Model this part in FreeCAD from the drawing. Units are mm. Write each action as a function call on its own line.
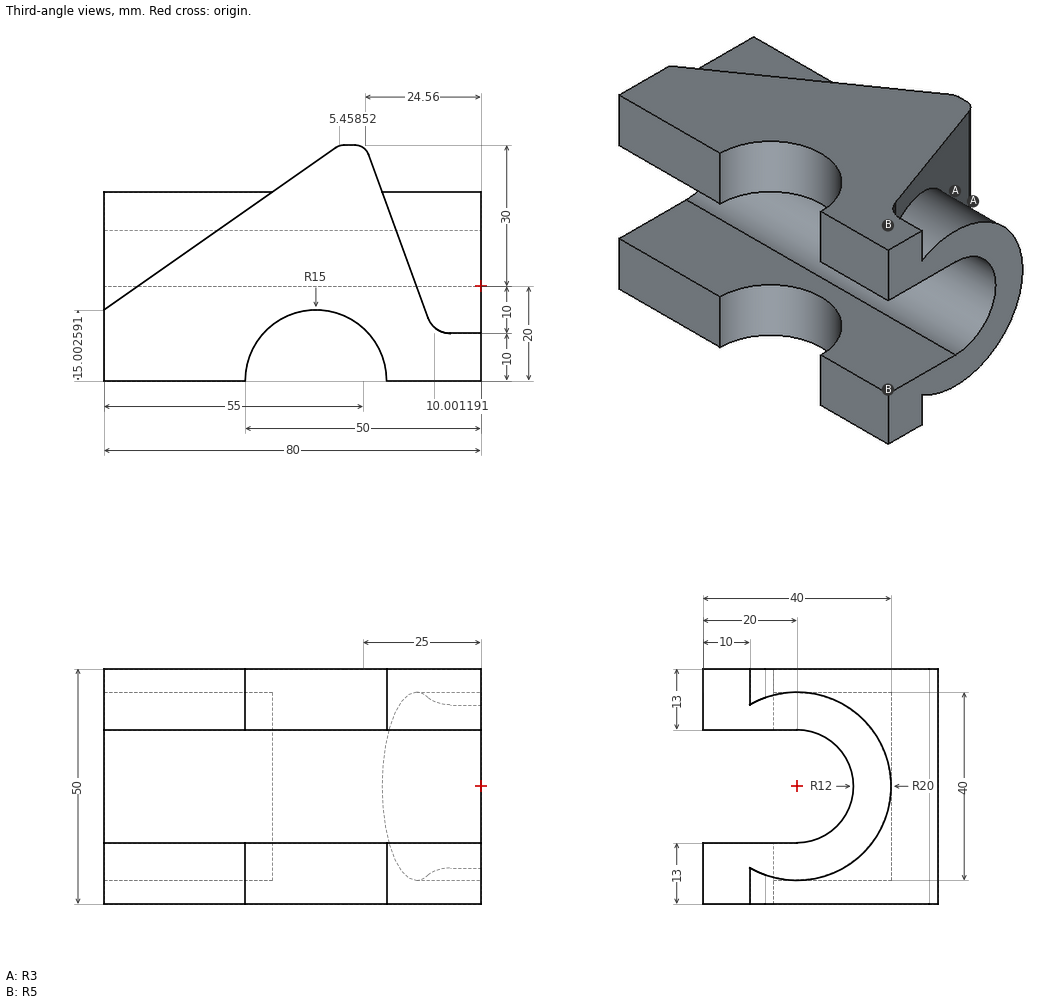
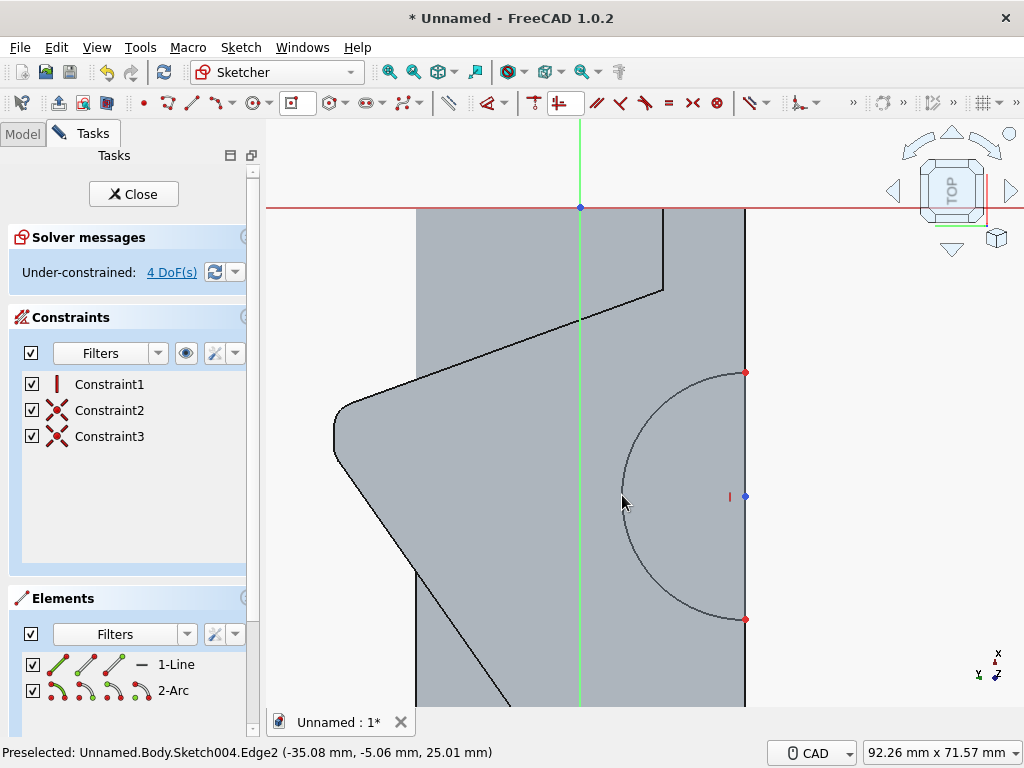
click(488, 104)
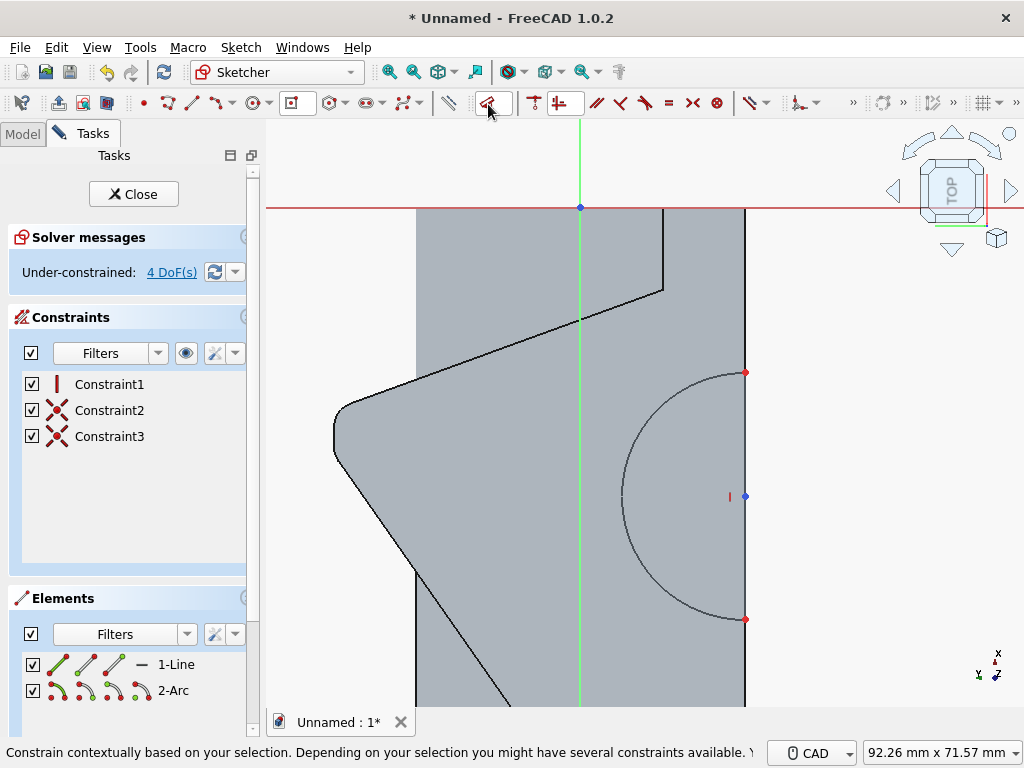
click(645, 424)
click(619, 405)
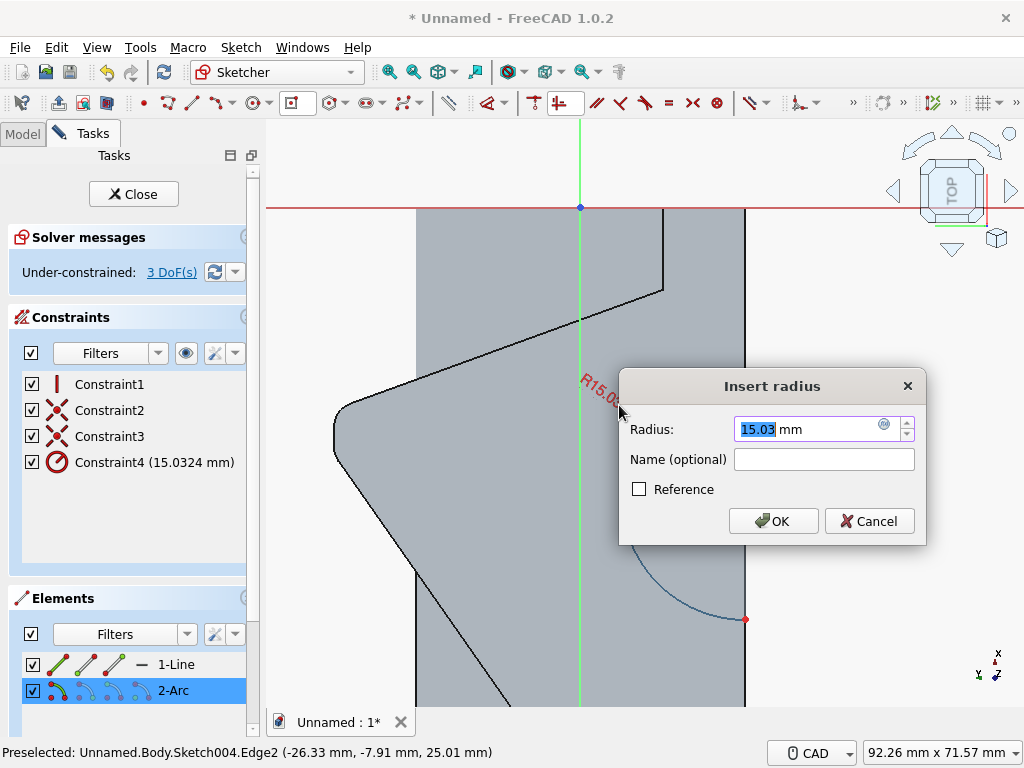
text(15)
key(Return)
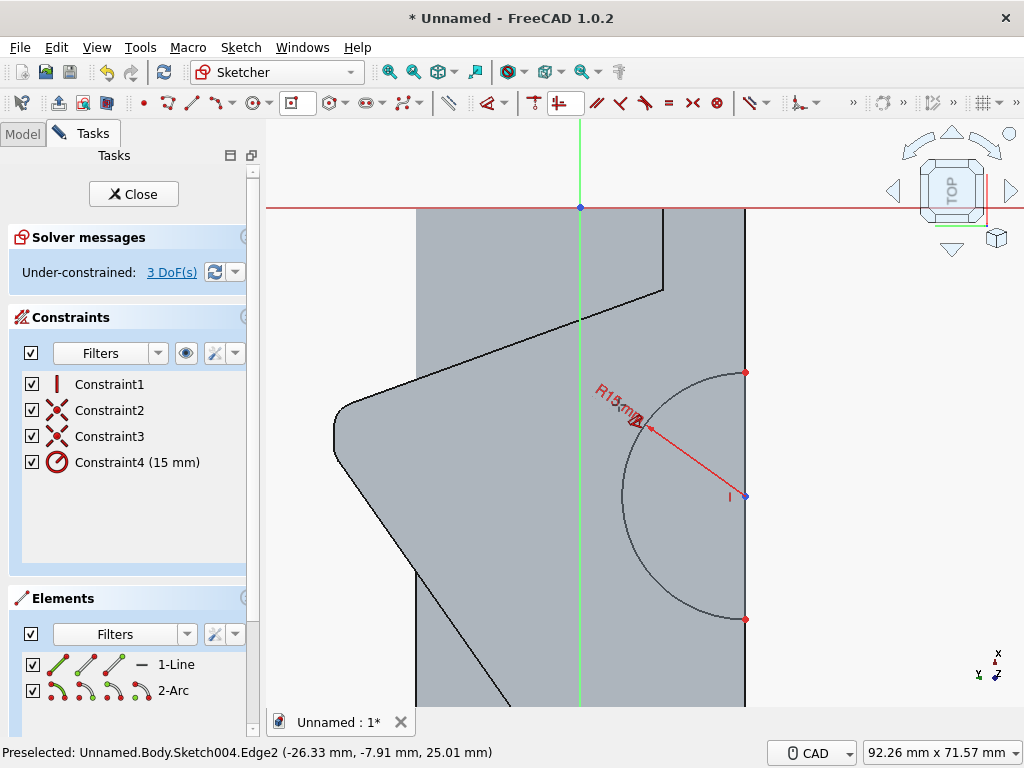
click(745, 619)
click(663, 653)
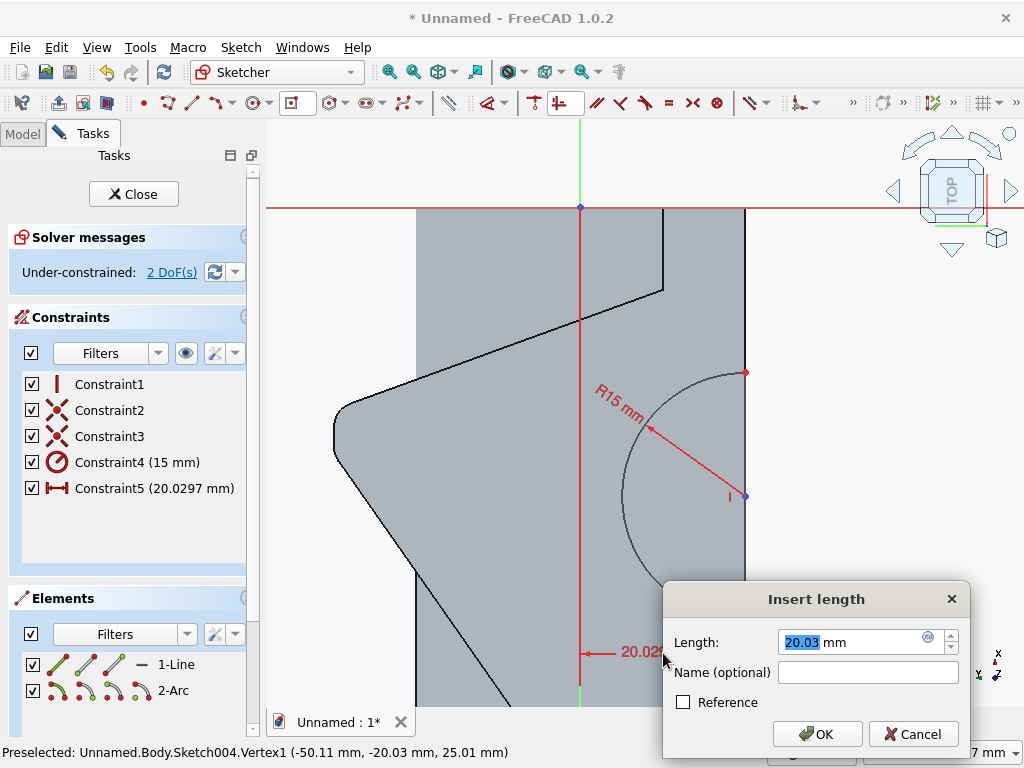
text(20)
key(Return)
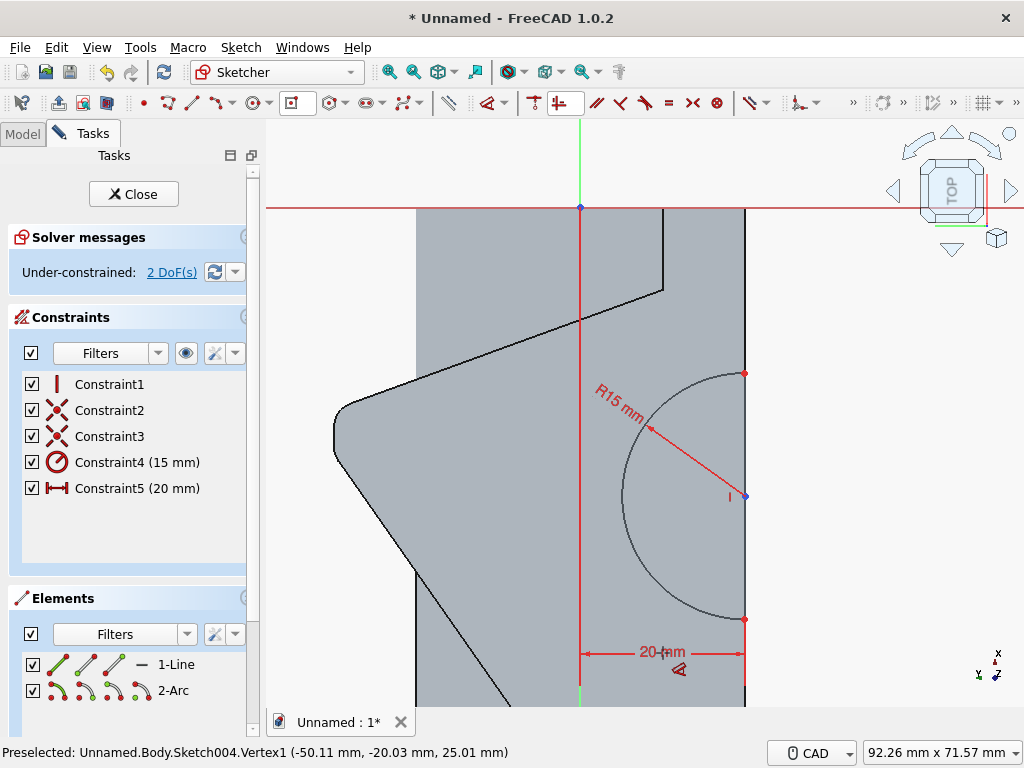
click(745, 619)
click(779, 414)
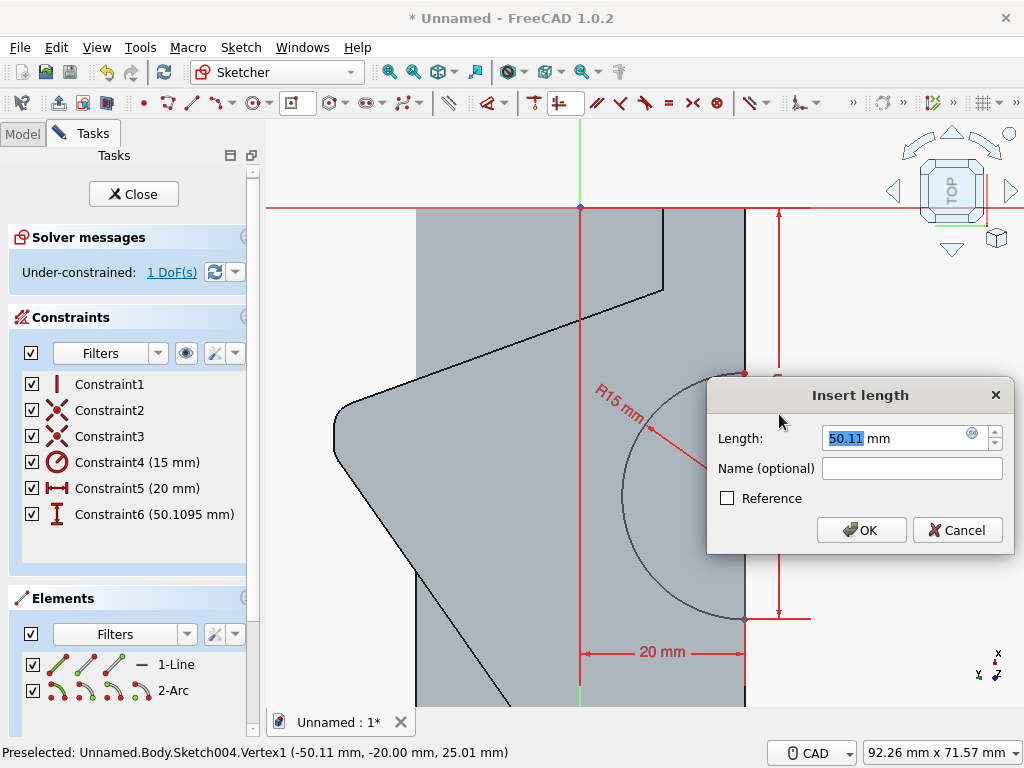
text(50)
key(Return)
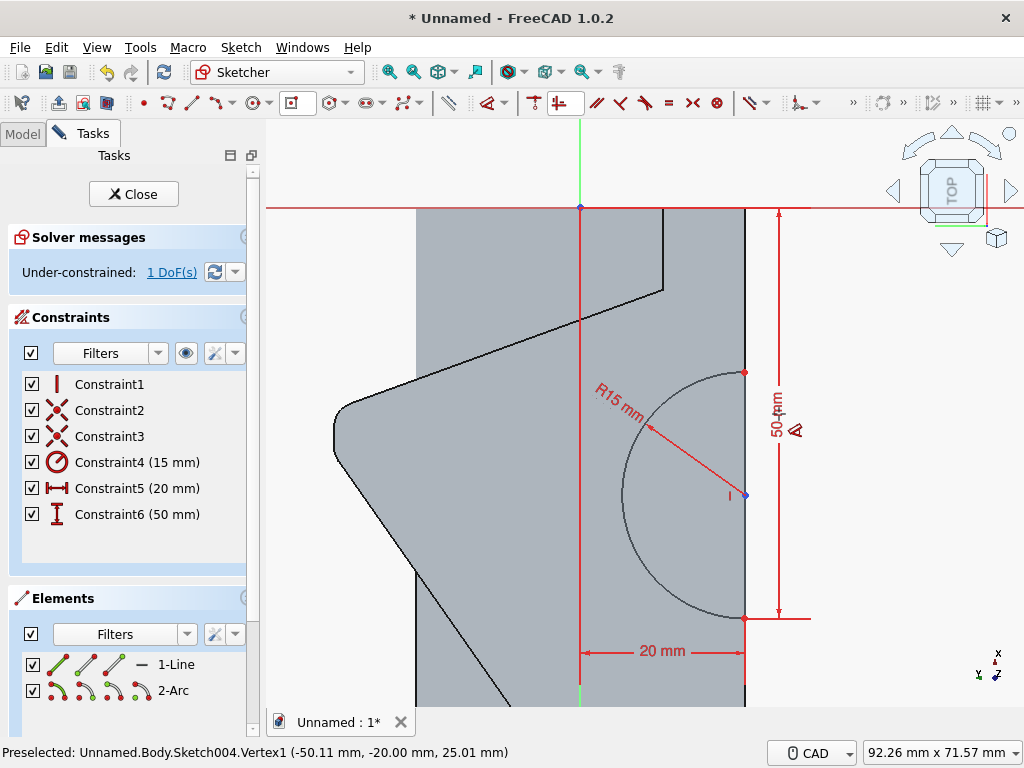
click(746, 495)
click(663, 174)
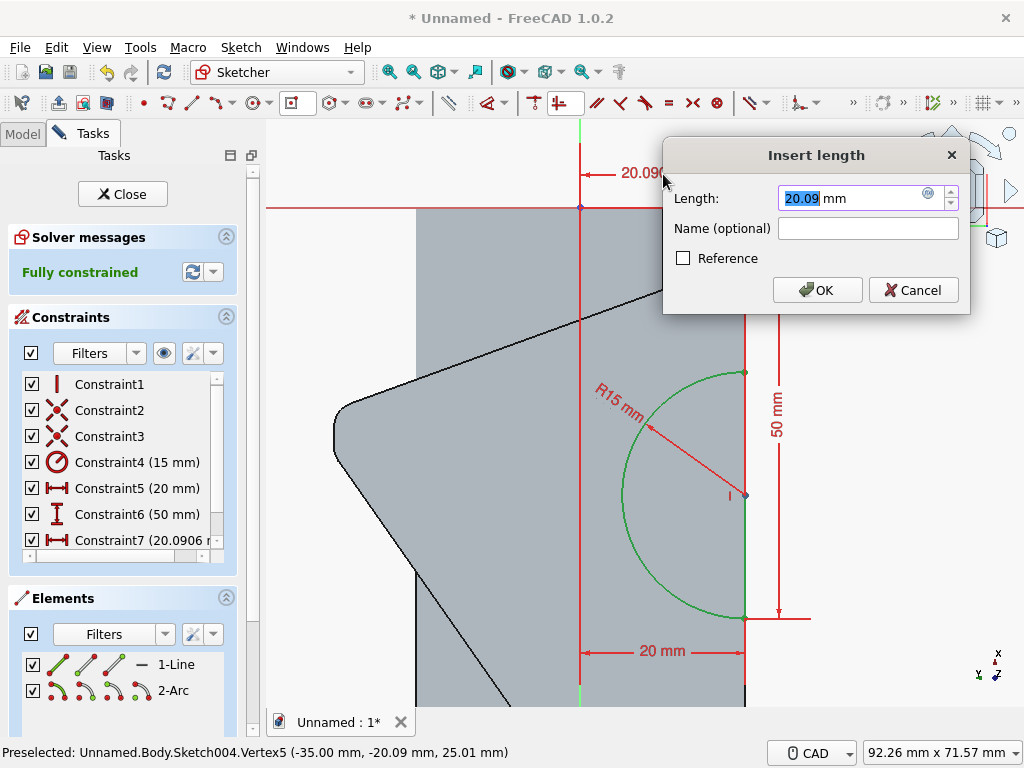
text(20)
key(Return)
key(Escape)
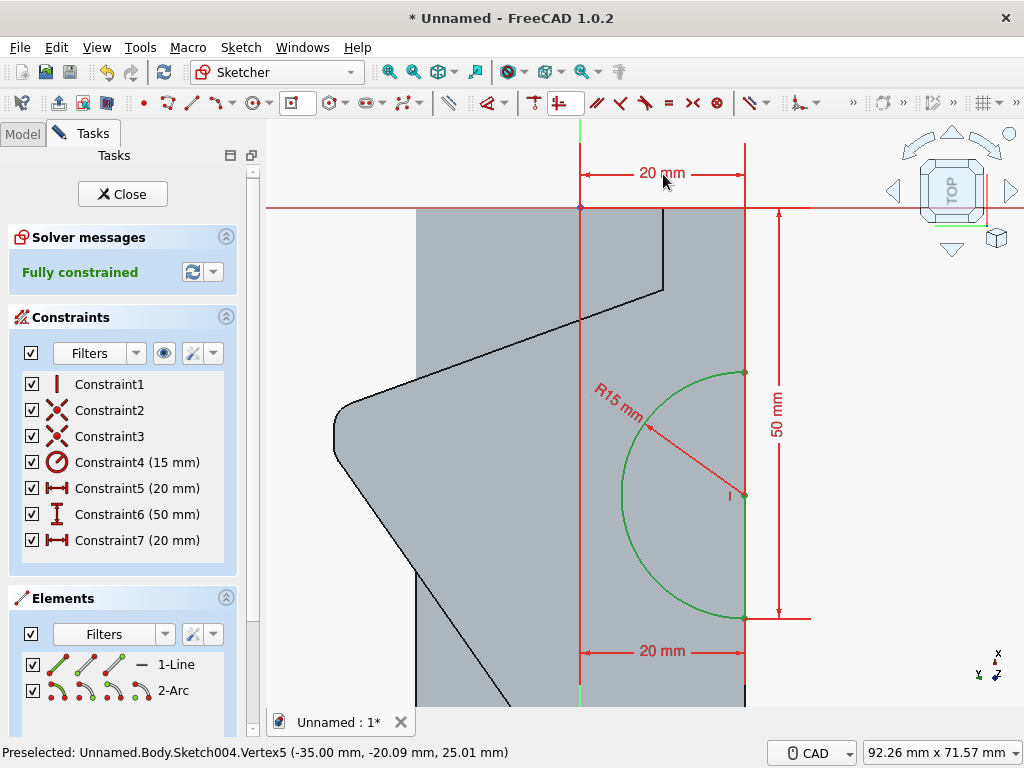
click(123, 194)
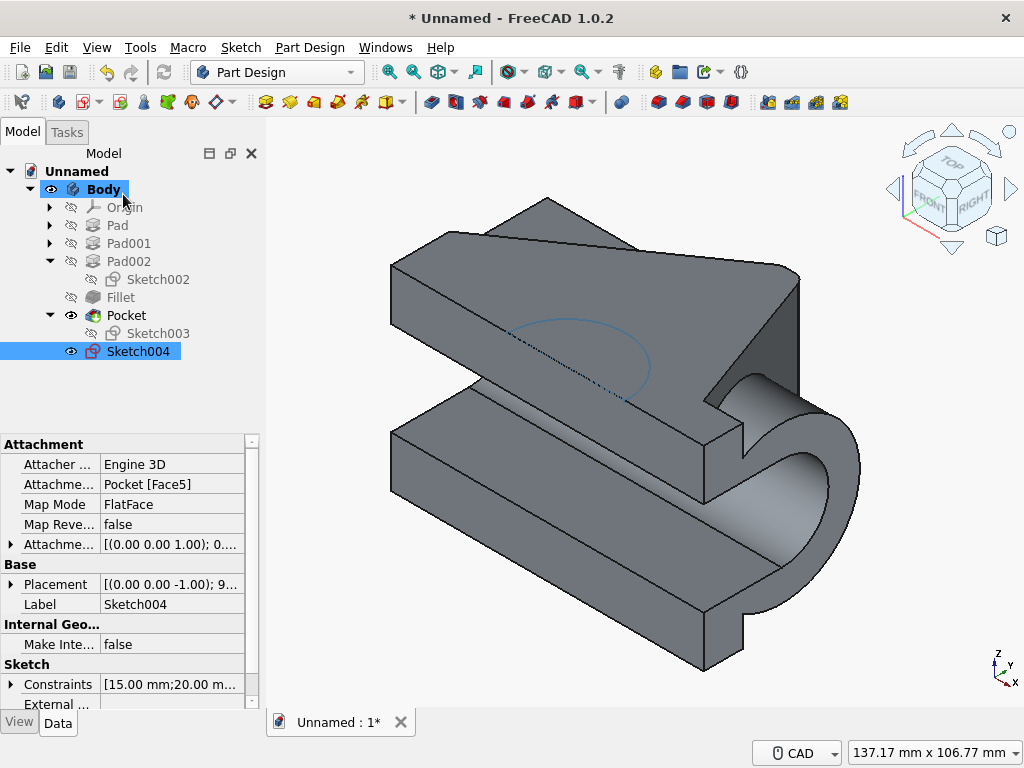
click(432, 102)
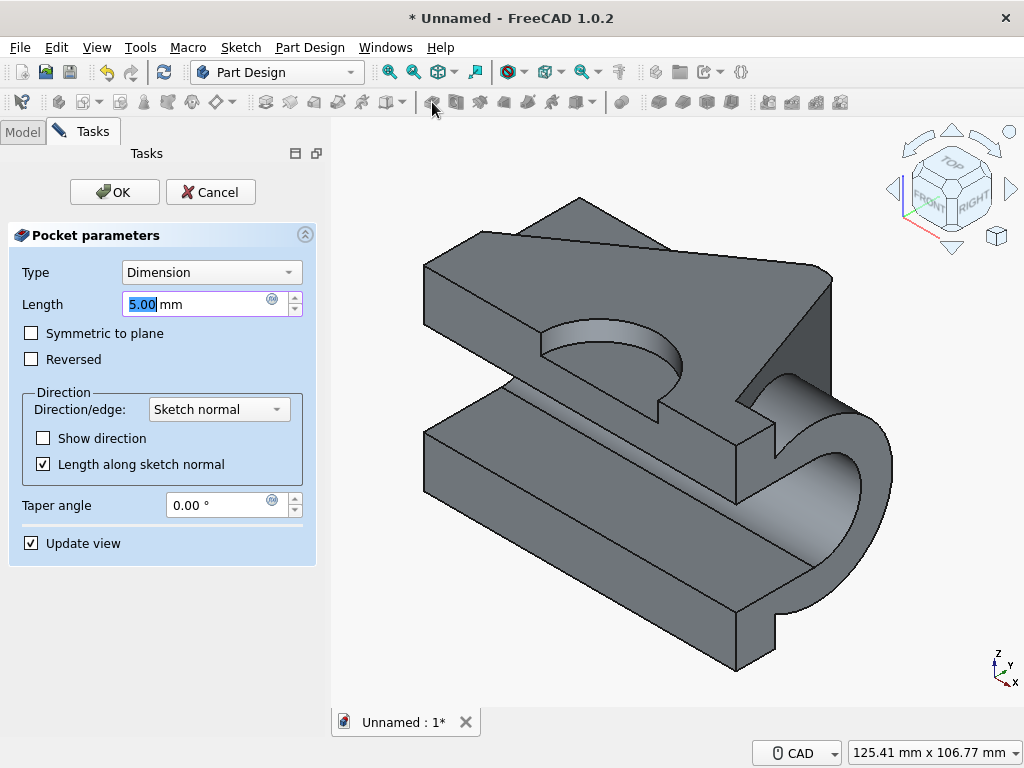
click(212, 272)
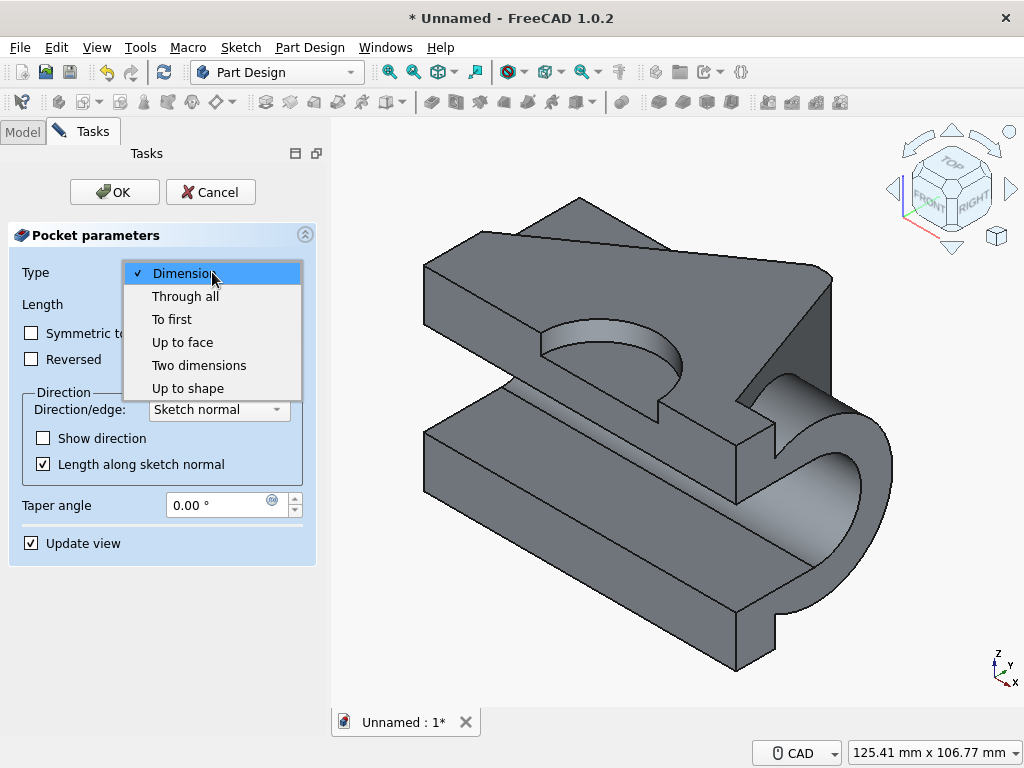
click(212, 296)